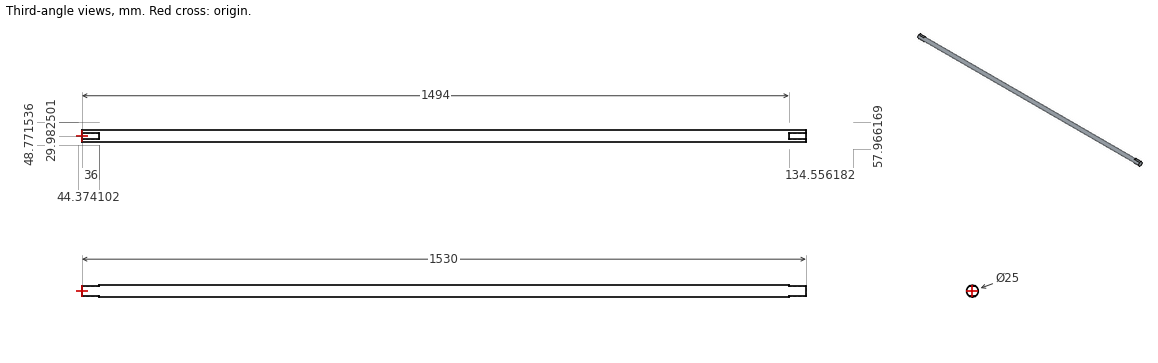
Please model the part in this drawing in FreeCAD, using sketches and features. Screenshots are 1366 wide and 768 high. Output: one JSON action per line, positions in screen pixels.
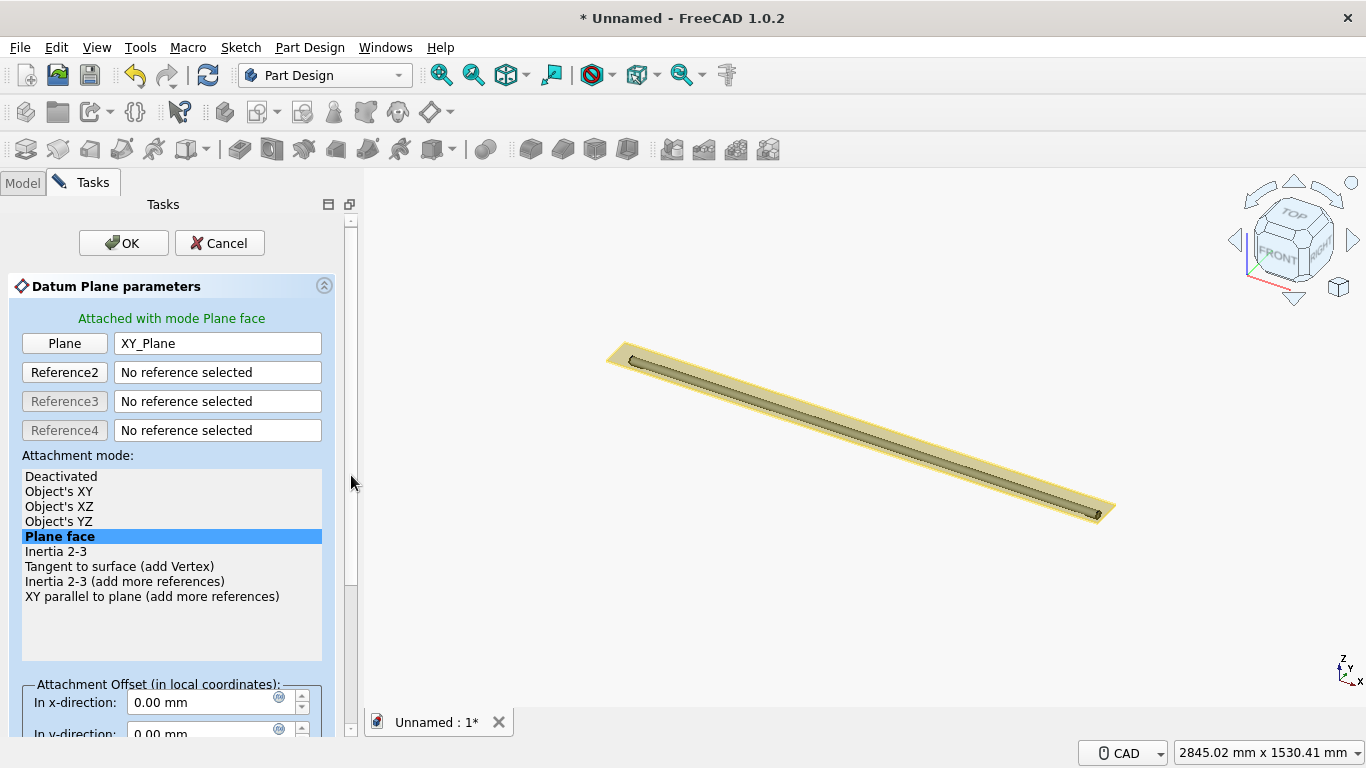
{"action": "left_click", "coordinate": [124, 243]}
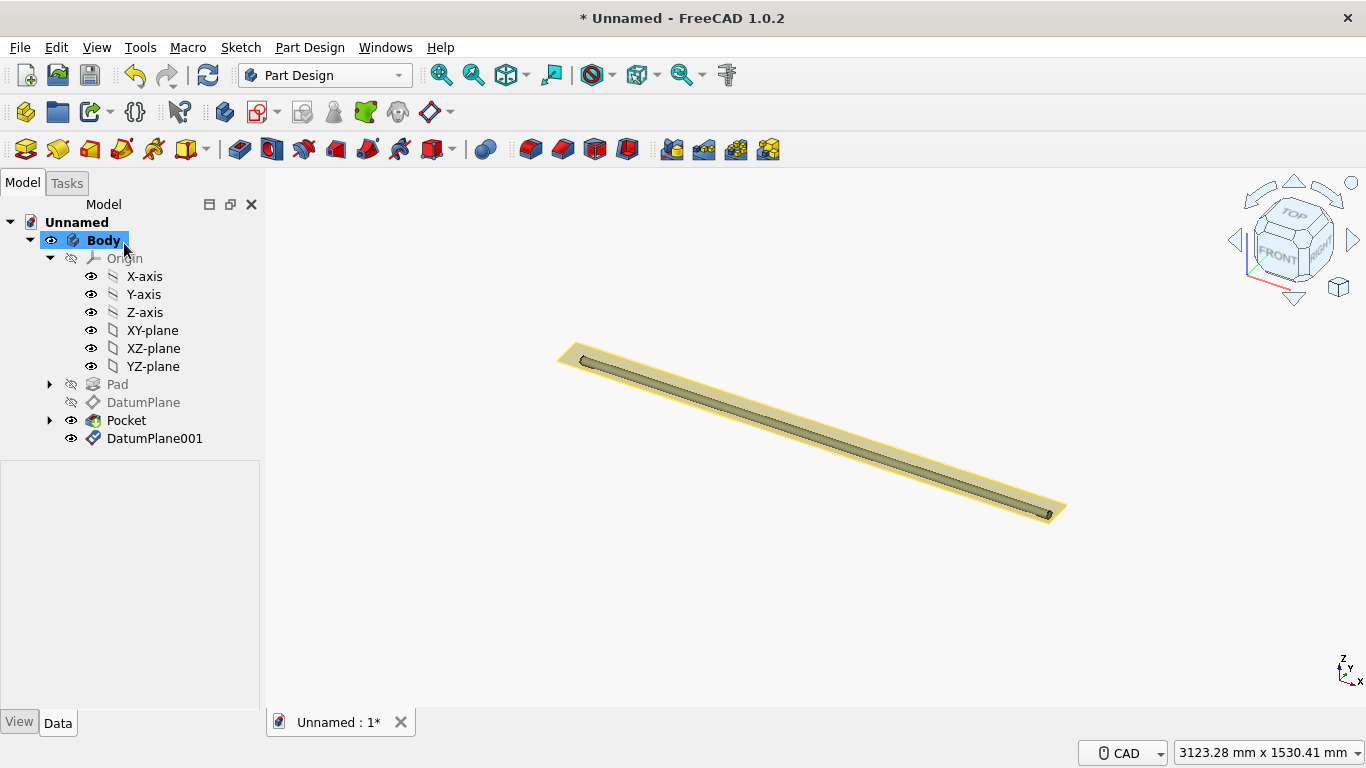
{"action": "left_click", "coordinate": [116, 438]}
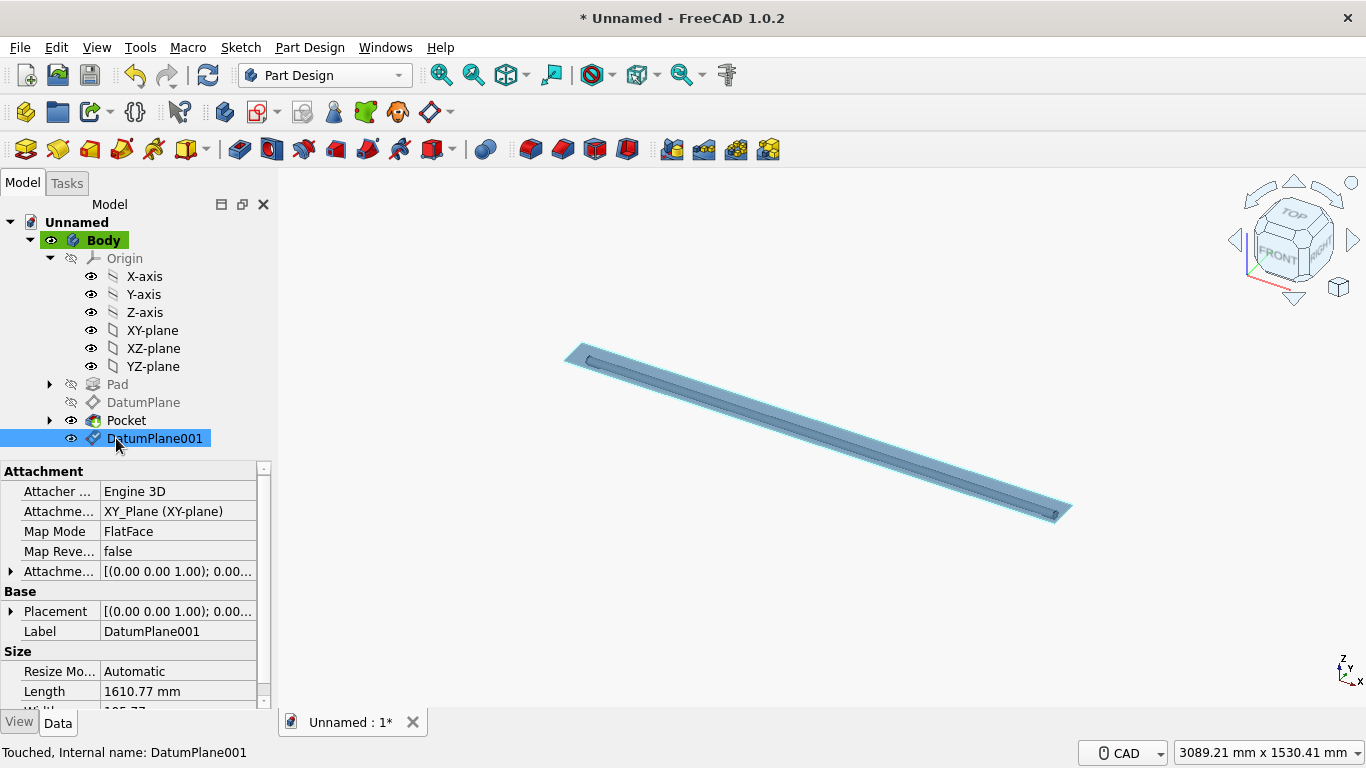
{"action": "left_click", "coordinate": [258, 112]}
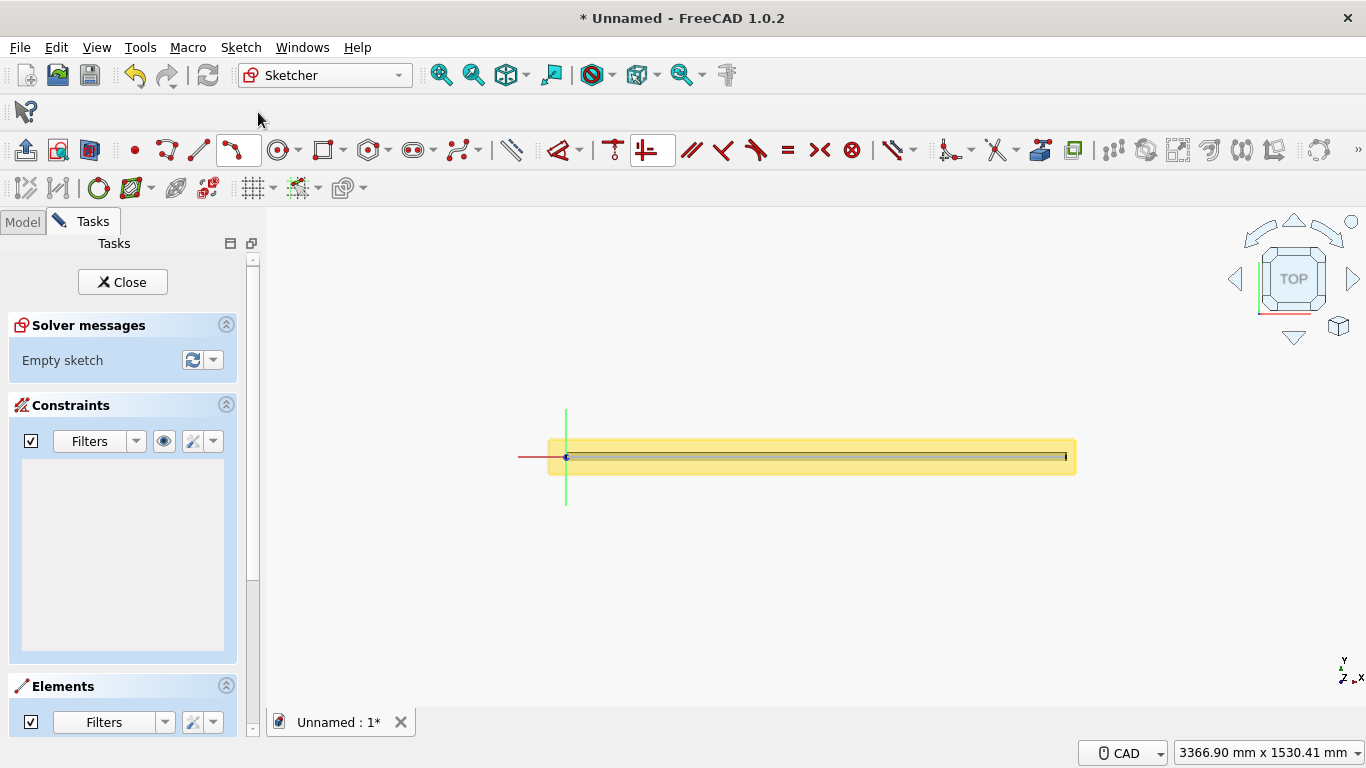
{"action": "left_click", "coordinate": [90, 150]}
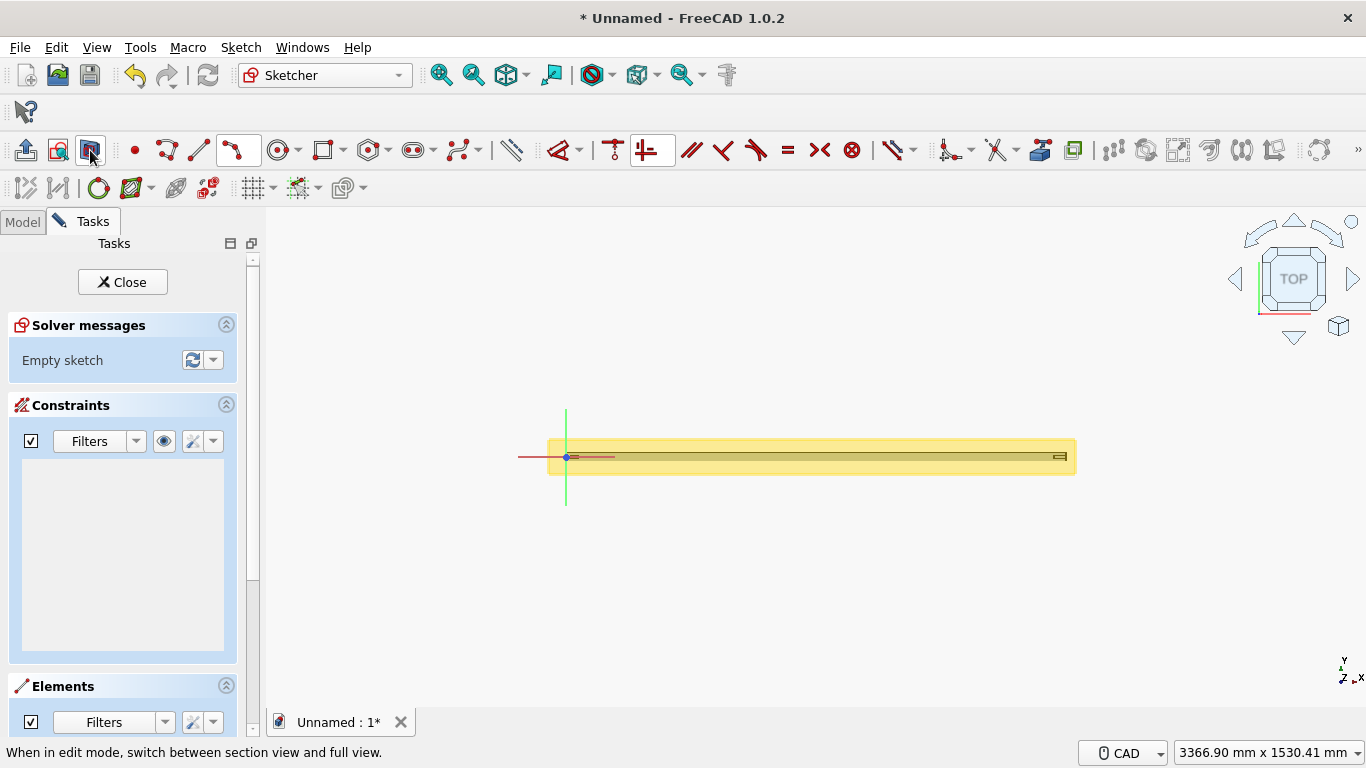
{"action": "left_click", "coordinate": [324, 150]}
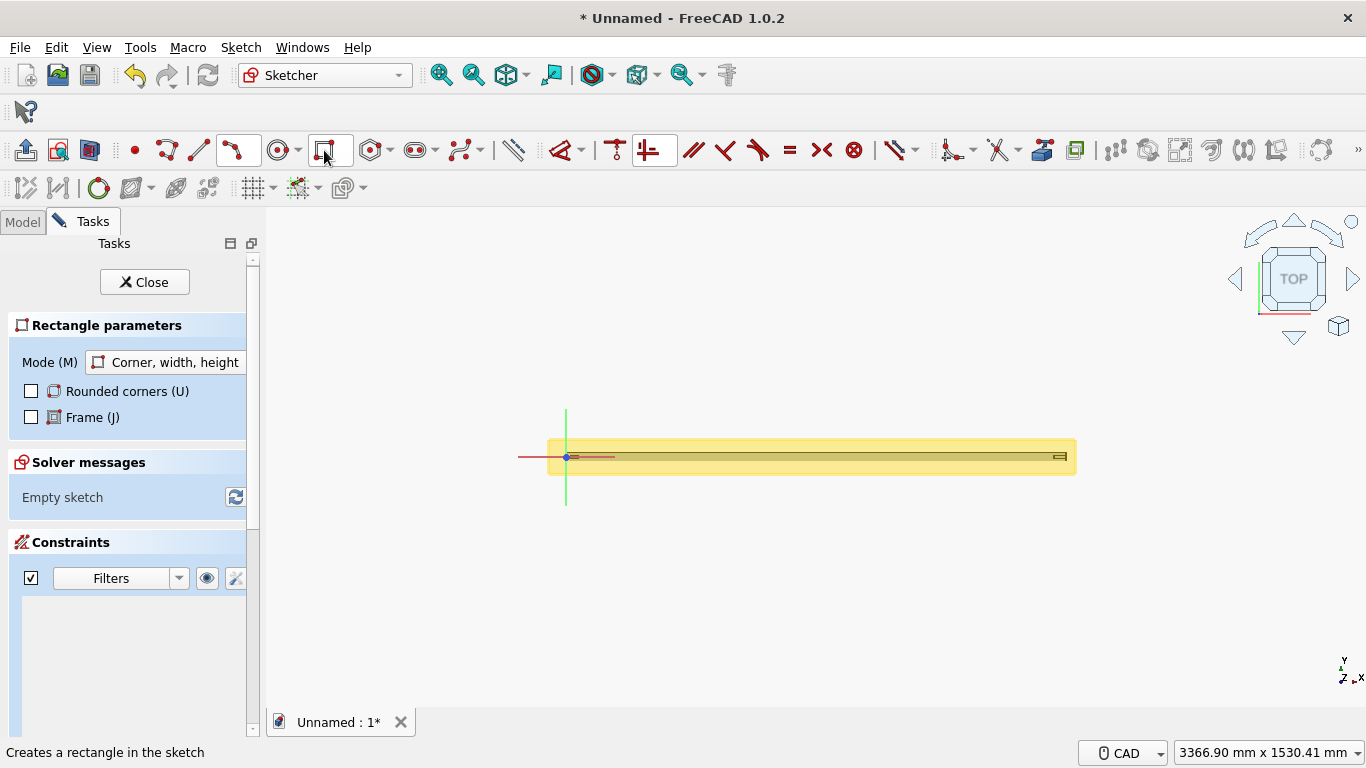
{"action": "scroll", "coordinate": [563, 447], "scroll_direction": "up", "scroll_amount": 9}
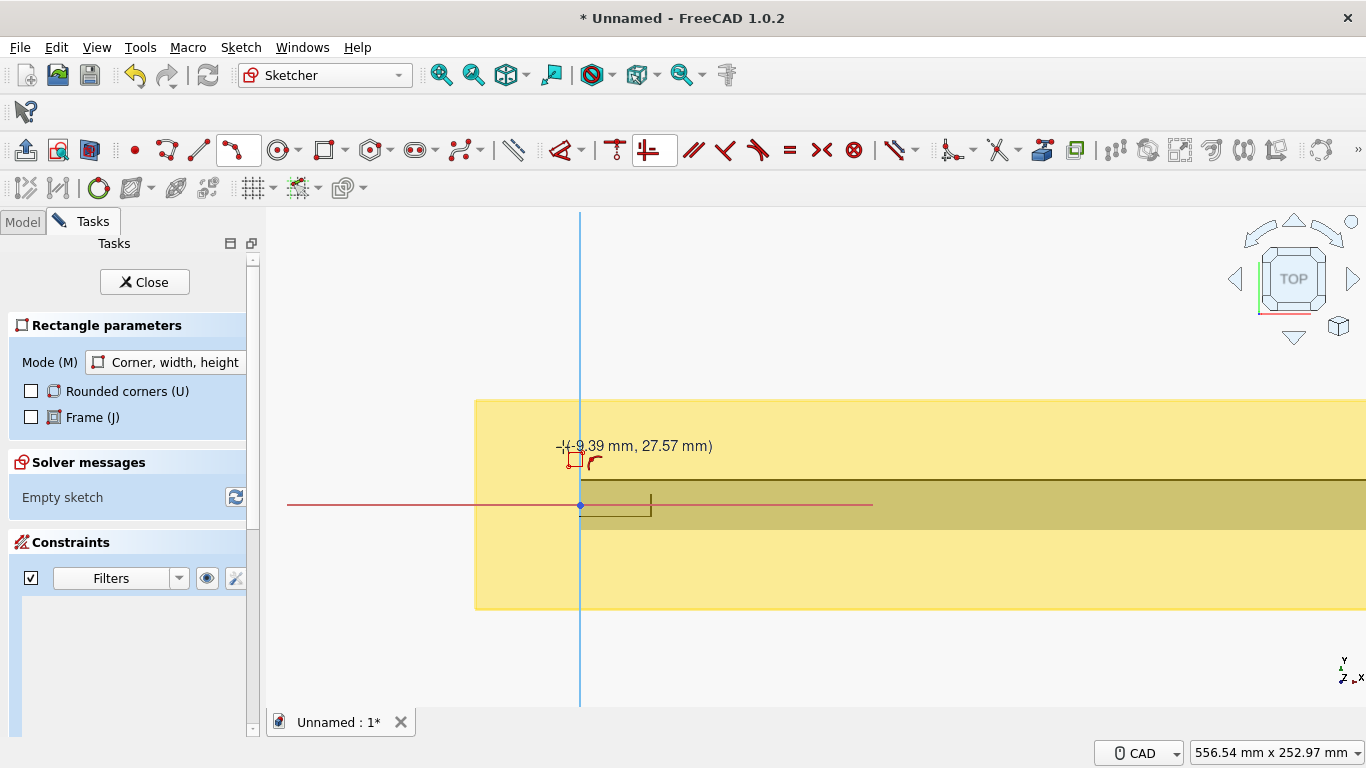
{"action": "left_click", "coordinate": [564, 446]}
{"action": "mouse_move", "coordinate": [651, 542]}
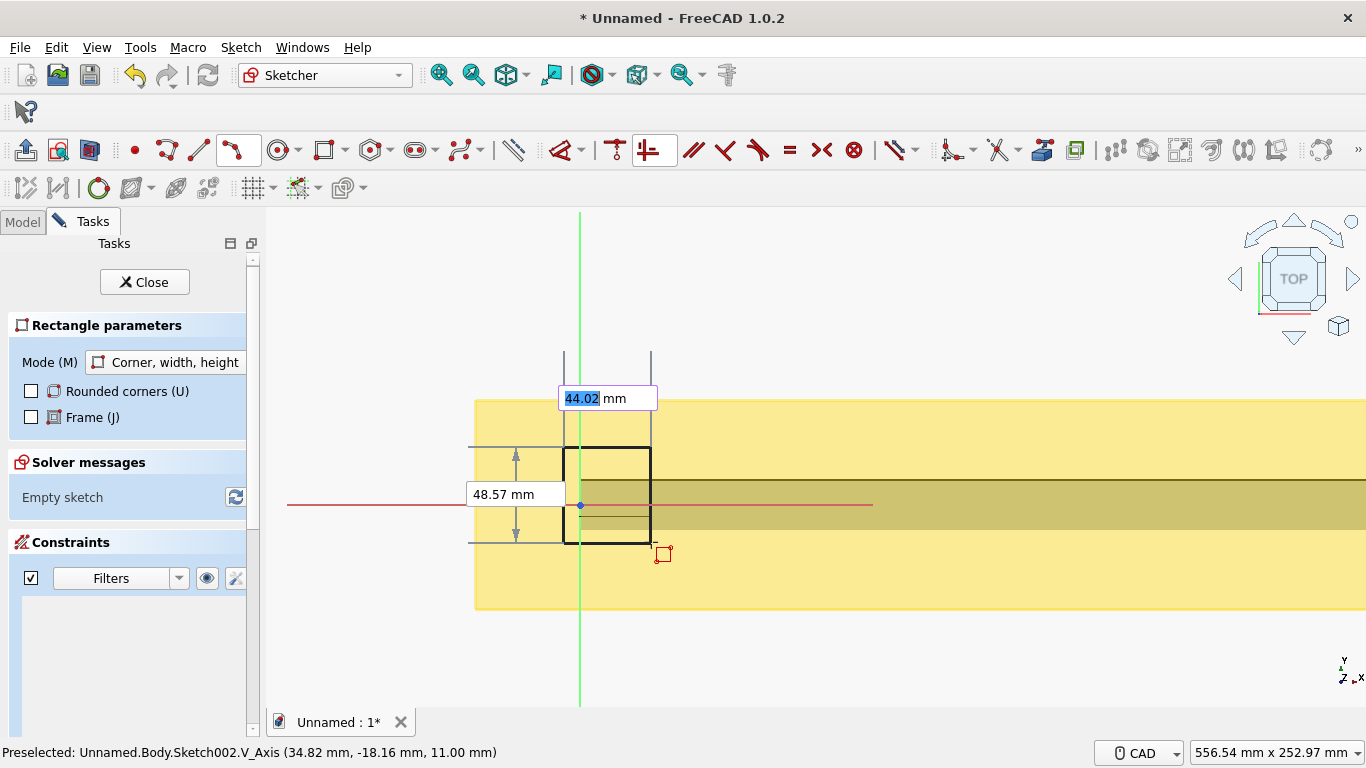
{"action": "type", "text": "44.374102"}
{"action": "key", "text": "Tab"}
{"action": "type", "text": "48.771536"}
{"action": "key", "text": "Return"}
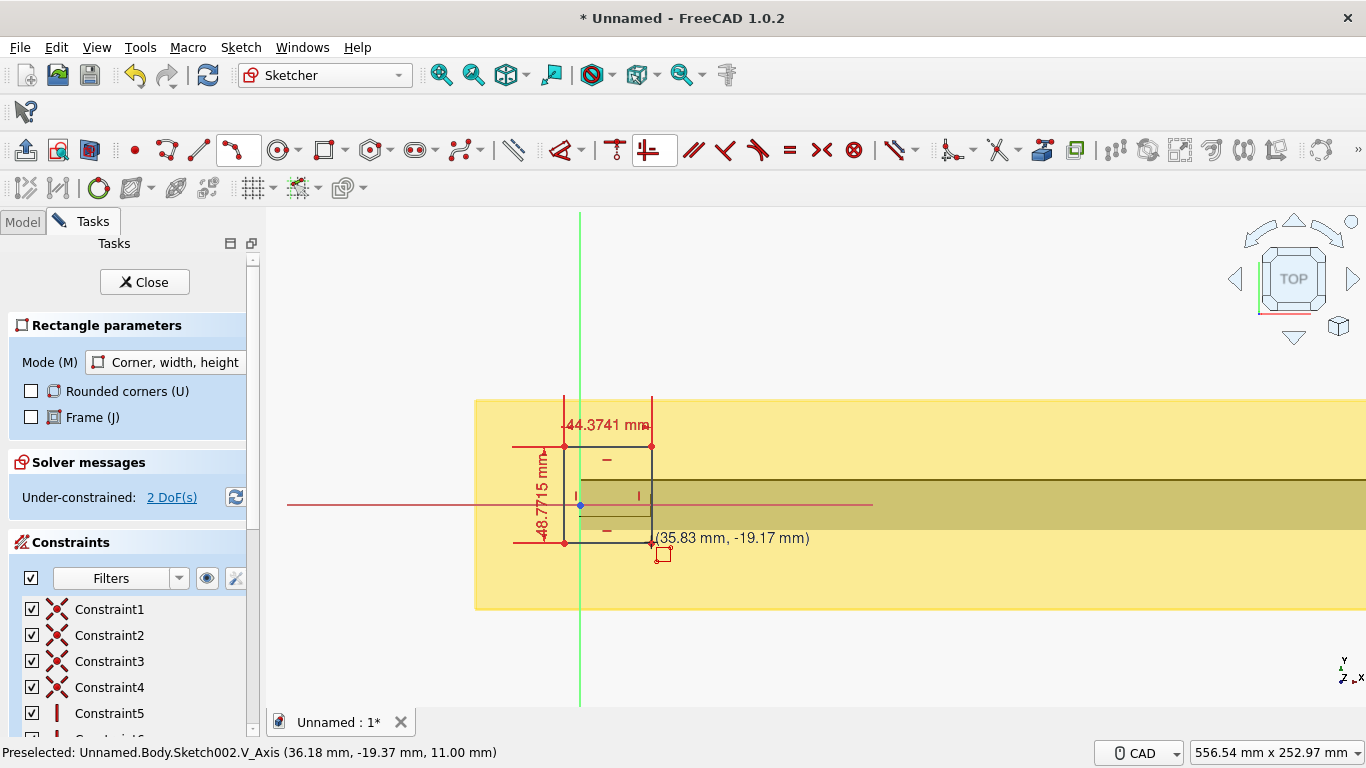
{"action": "scroll", "coordinate": [385, 445], "scroll_direction": "down", "scroll_amount": 8}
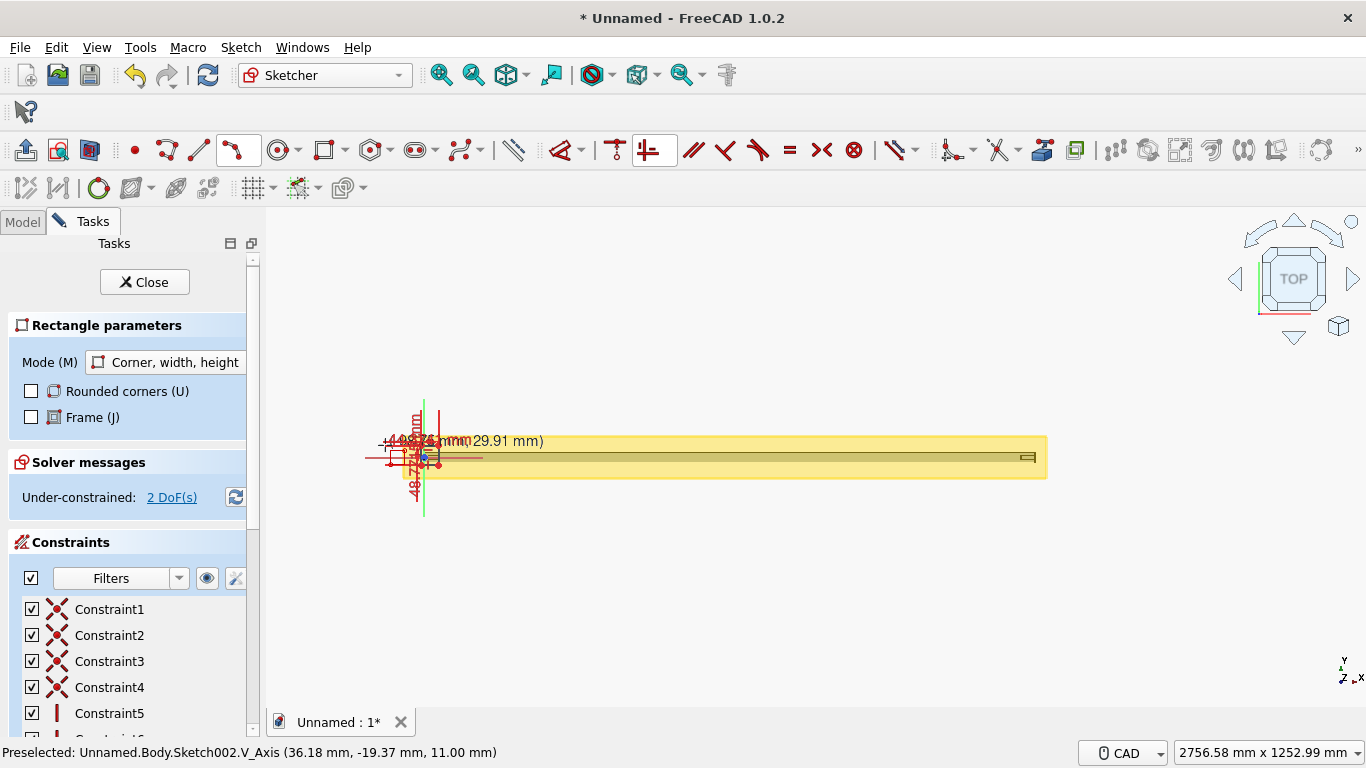
{"action": "scroll", "coordinate": [1021, 446], "scroll_direction": "up", "scroll_amount": 2}